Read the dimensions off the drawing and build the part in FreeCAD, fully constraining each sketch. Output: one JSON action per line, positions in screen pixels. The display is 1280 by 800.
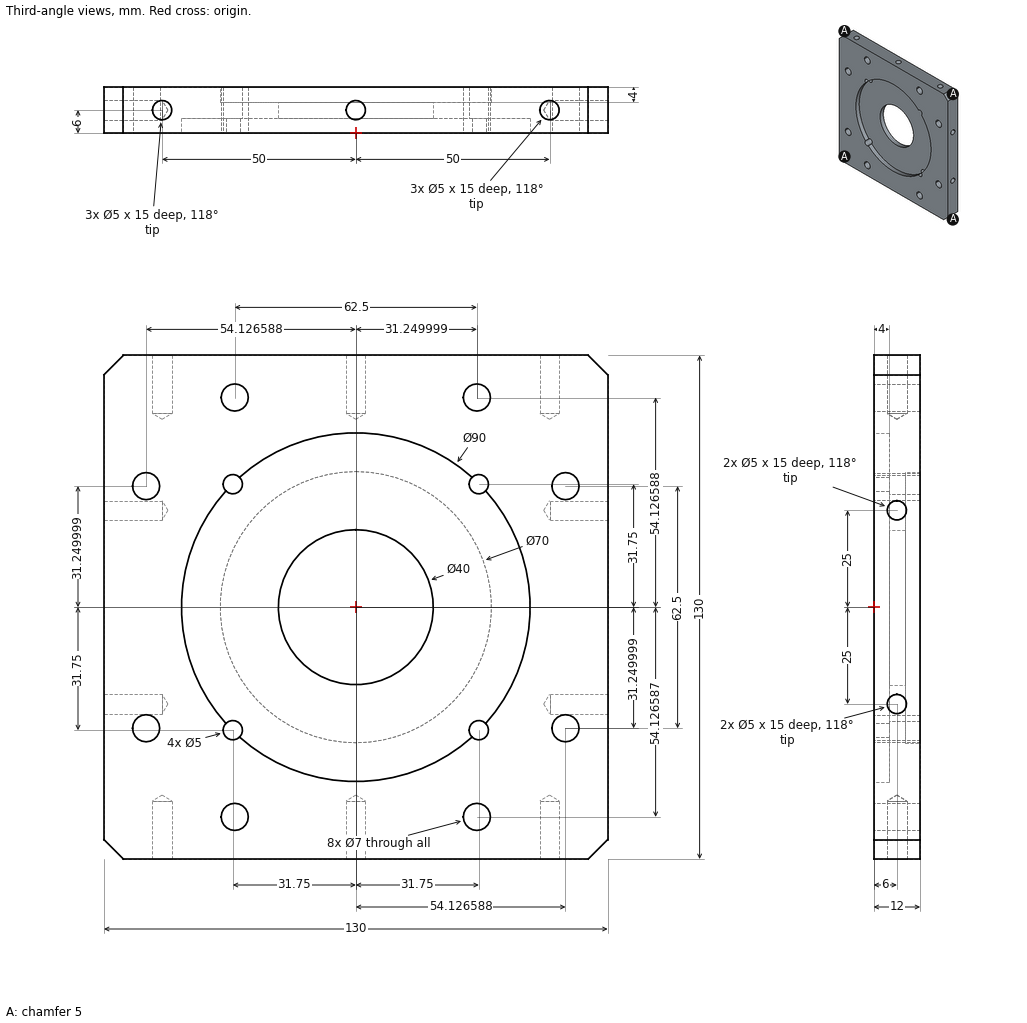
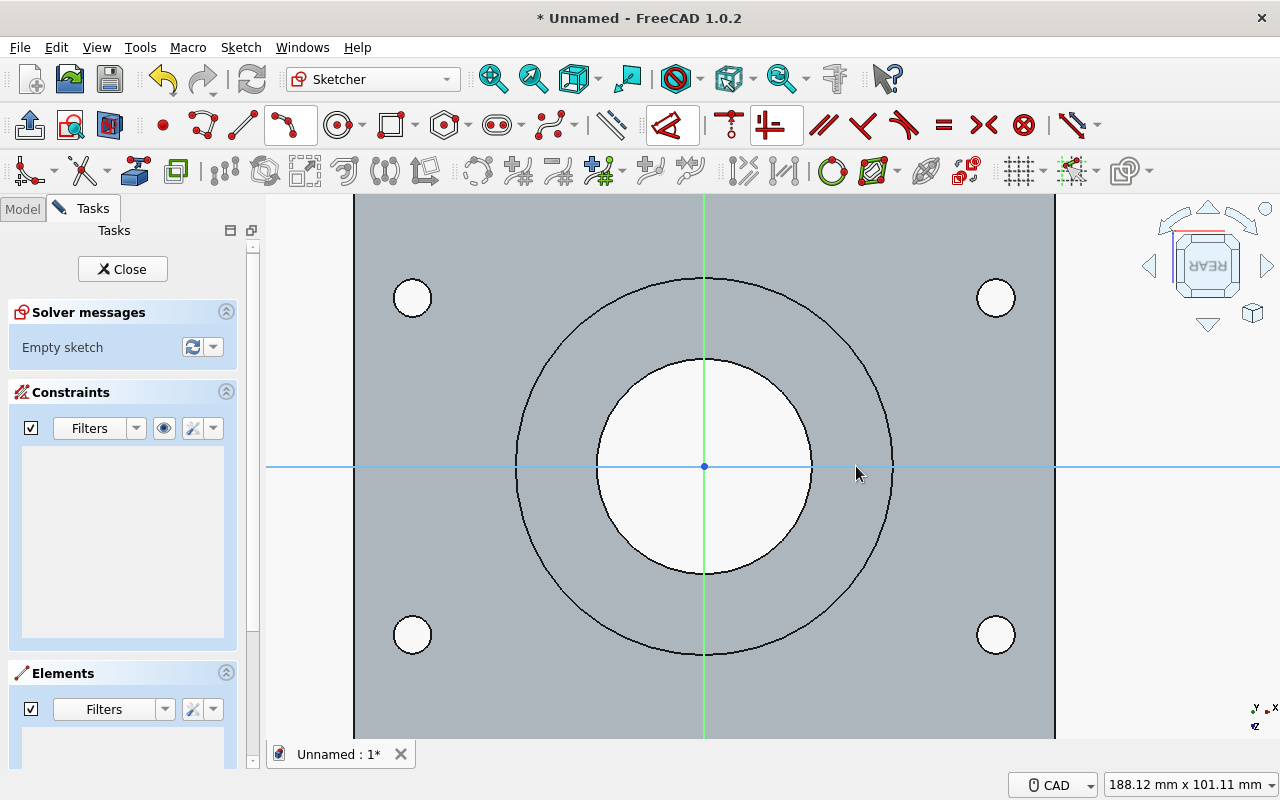
{"action": "key", "text": "g c"}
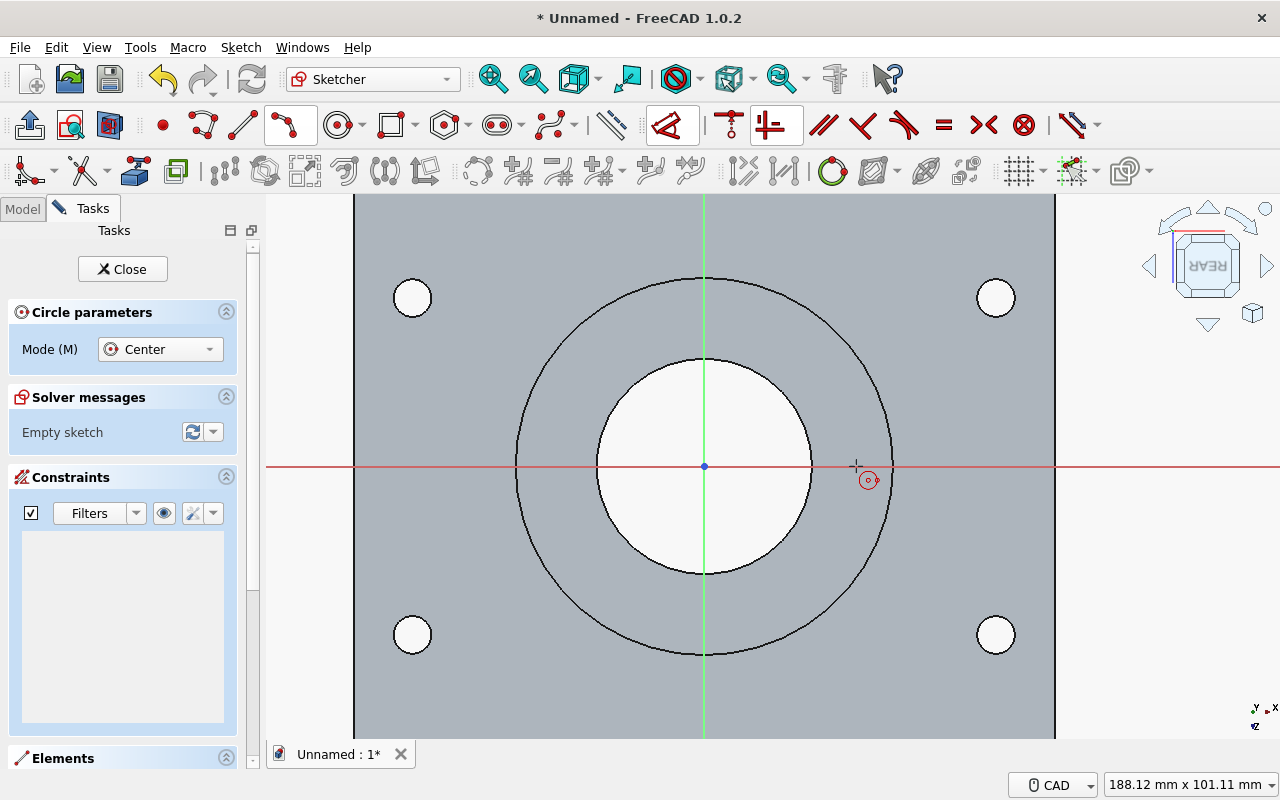
{"action": "scroll", "coordinate": [533, 295], "scroll_direction": "up", "scroll_amount": 3}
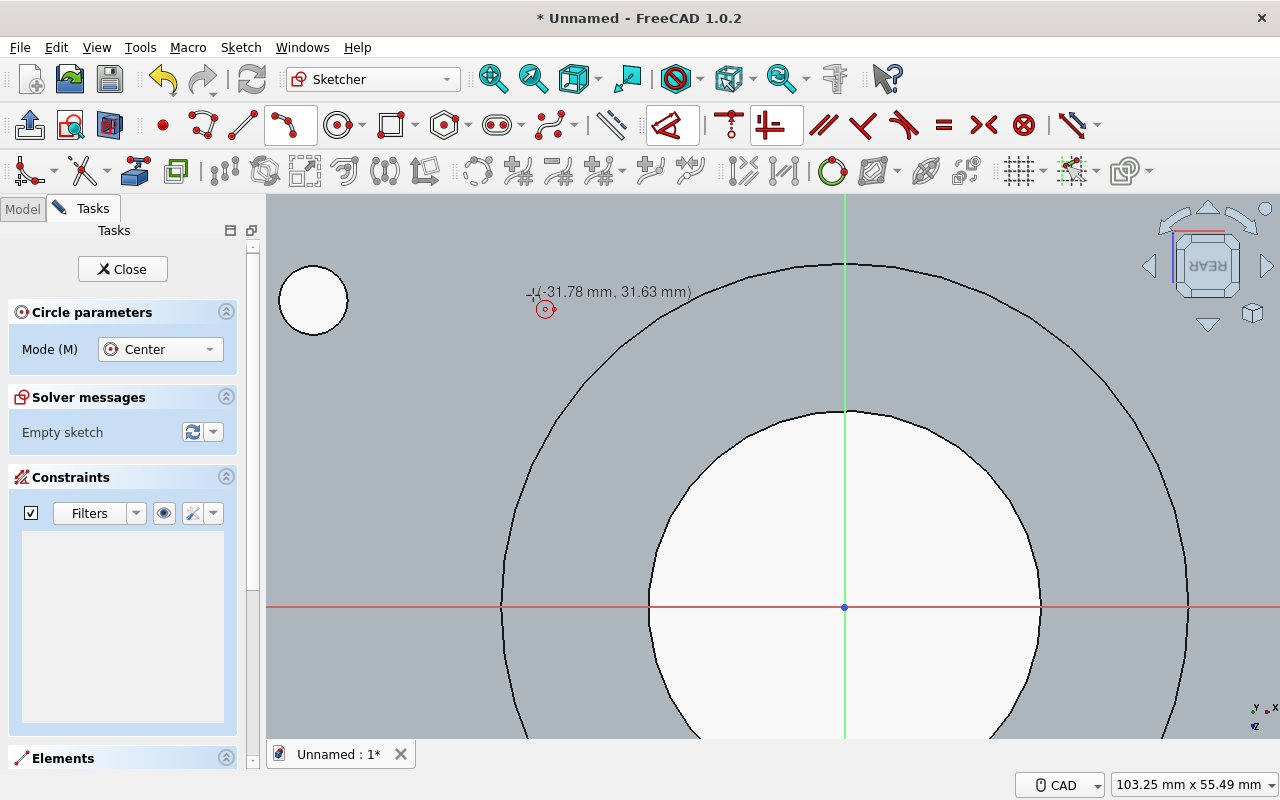
{"action": "left_click", "coordinate": [533, 296]}
{"action": "left_click", "coordinate": [550, 278]}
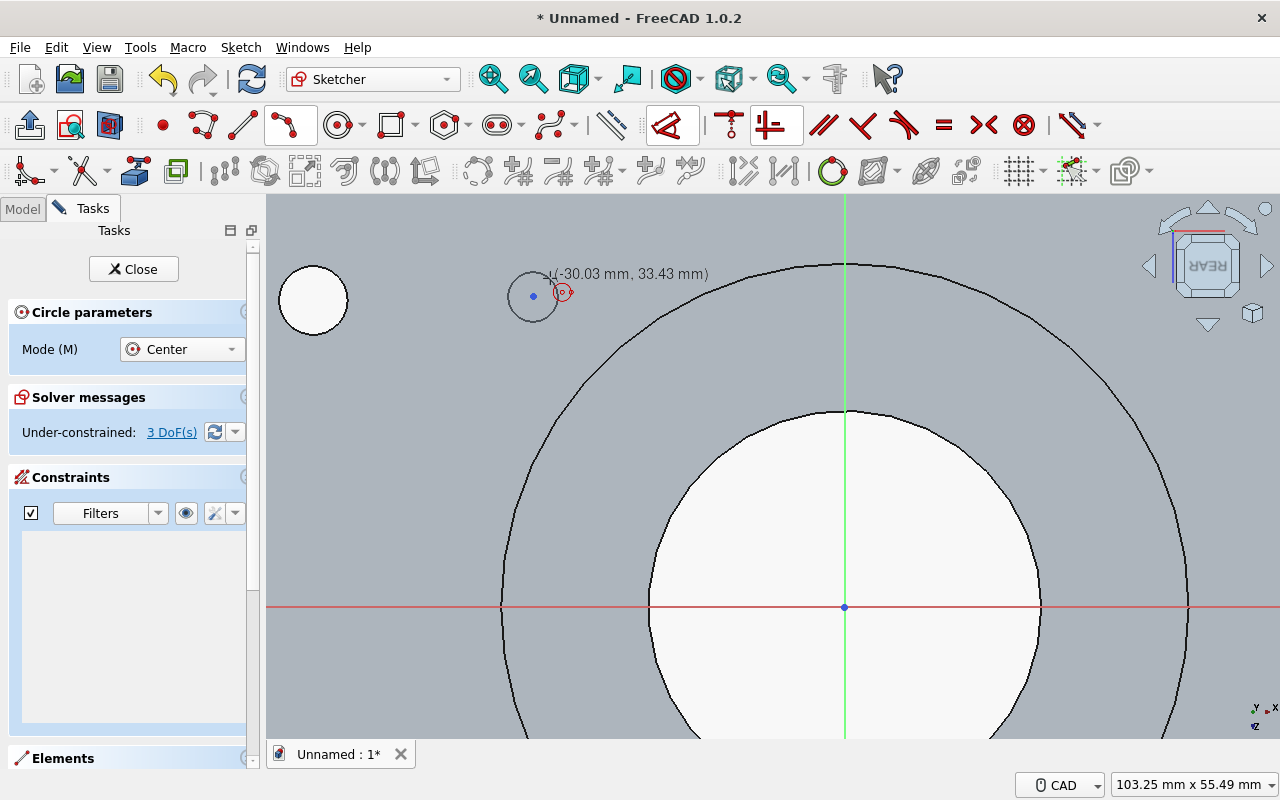
{"action": "scroll", "coordinate": [534, 295], "scroll_direction": "down", "scroll_amount": 3}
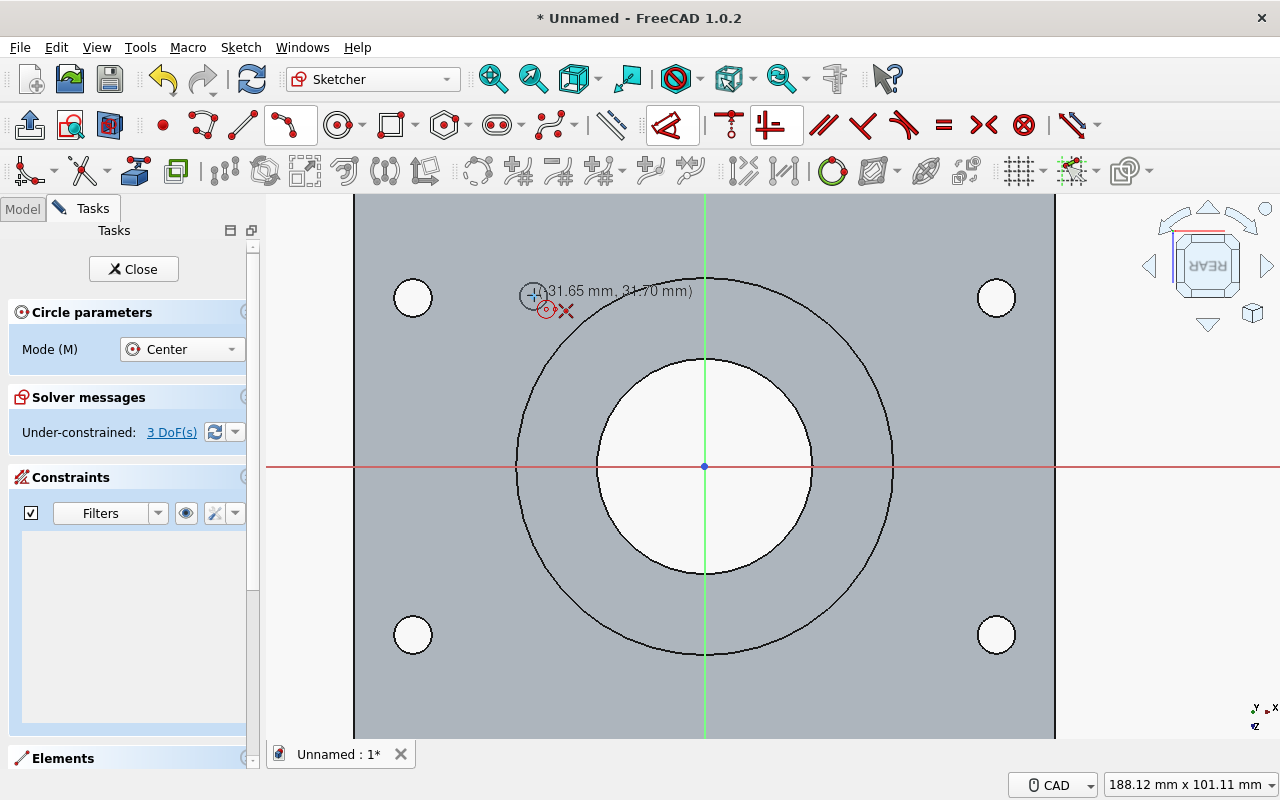
{"action": "scroll", "coordinate": [876, 295], "scroll_direction": "up", "scroll_amount": 3}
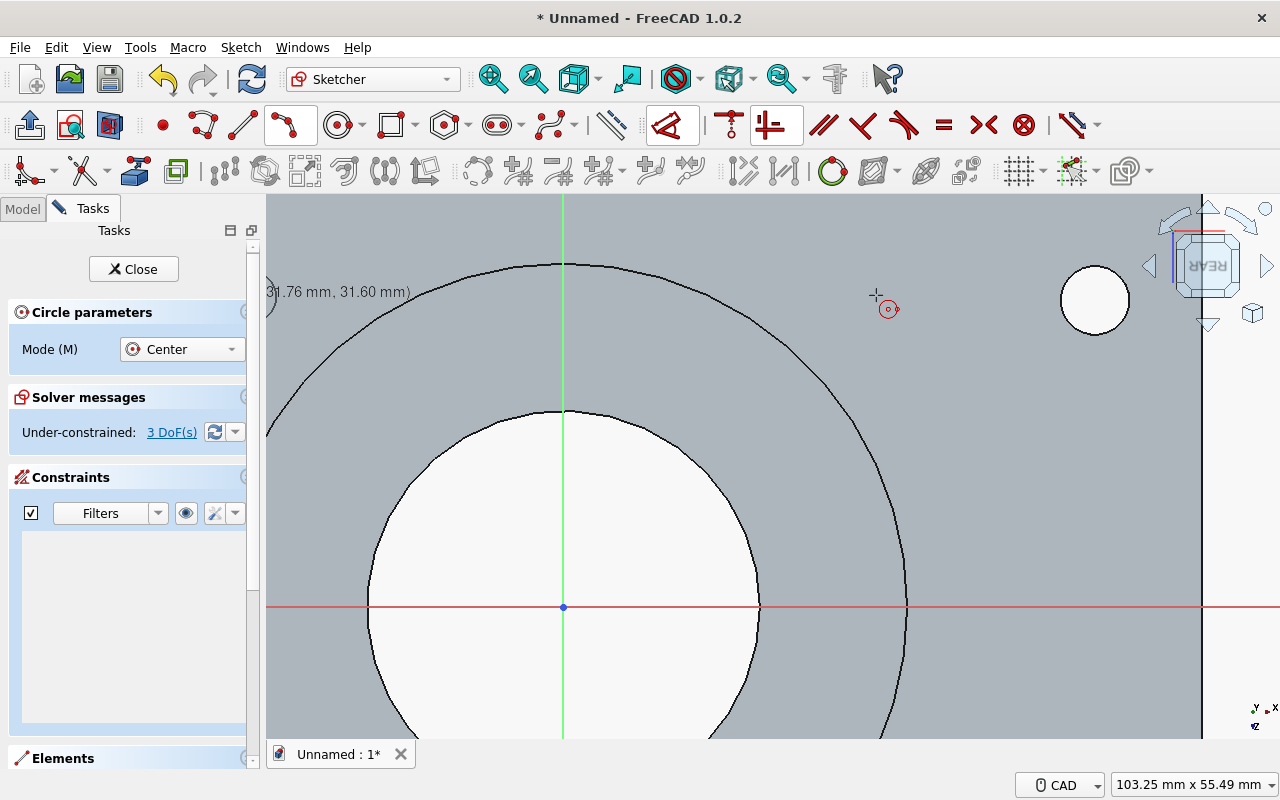
{"action": "left_click", "coordinate": [875, 296]}
{"action": "left_click", "coordinate": [893, 278]}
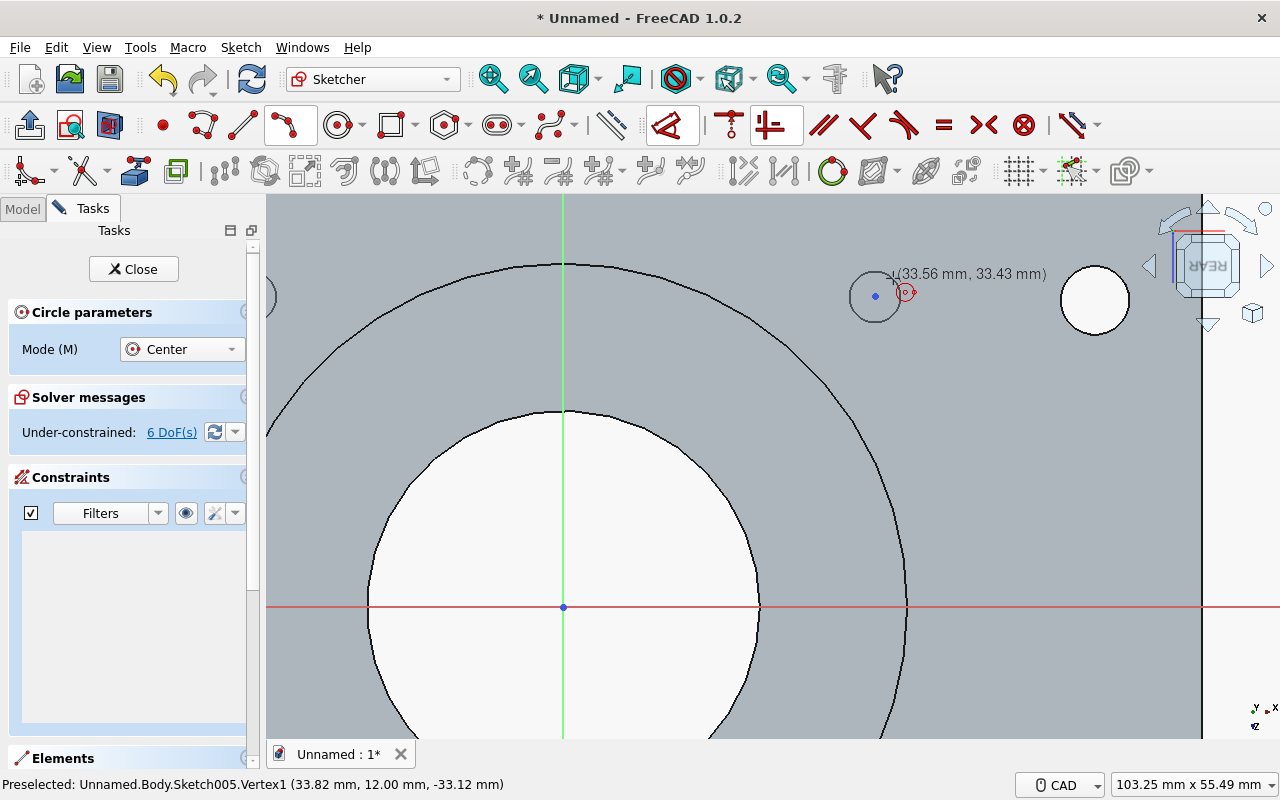
{"action": "scroll", "coordinate": [876, 295], "scroll_direction": "down", "scroll_amount": 3}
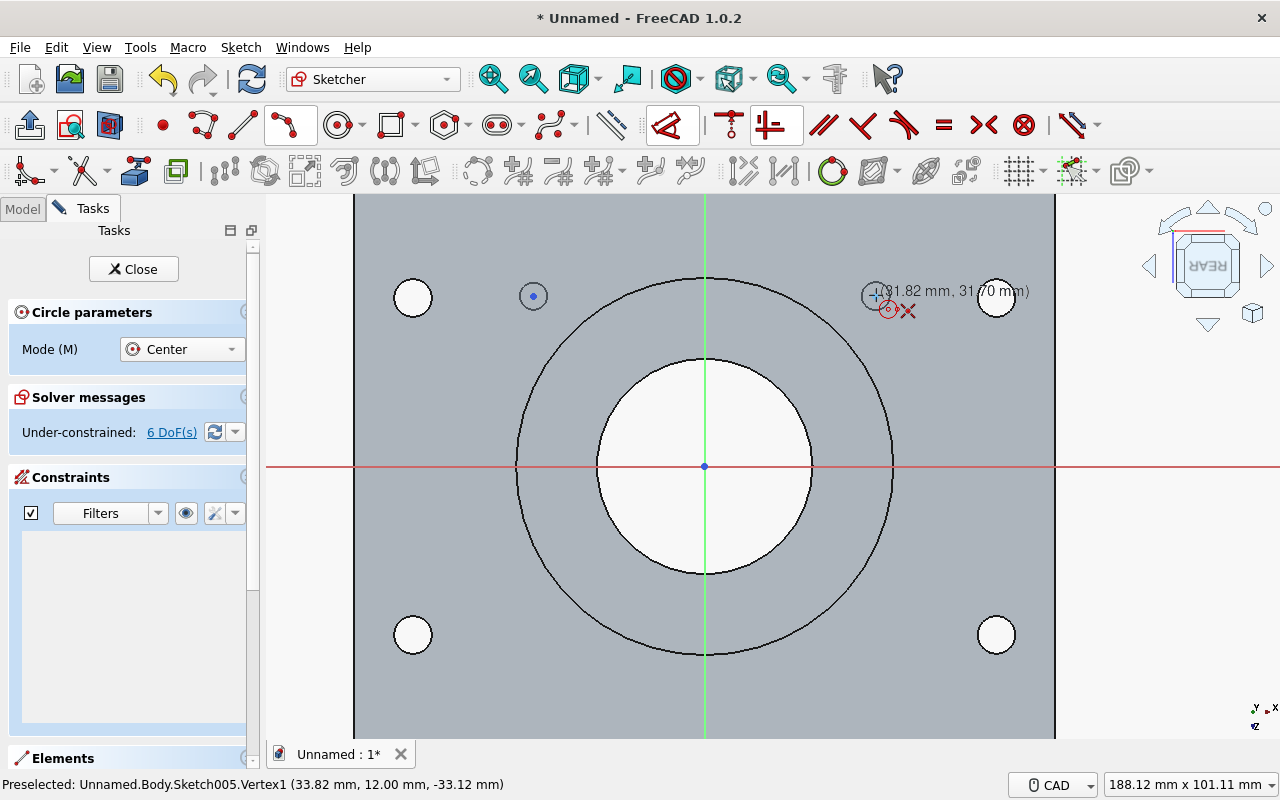
{"action": "scroll", "coordinate": [876, 638], "scroll_direction": "up", "scroll_amount": 3}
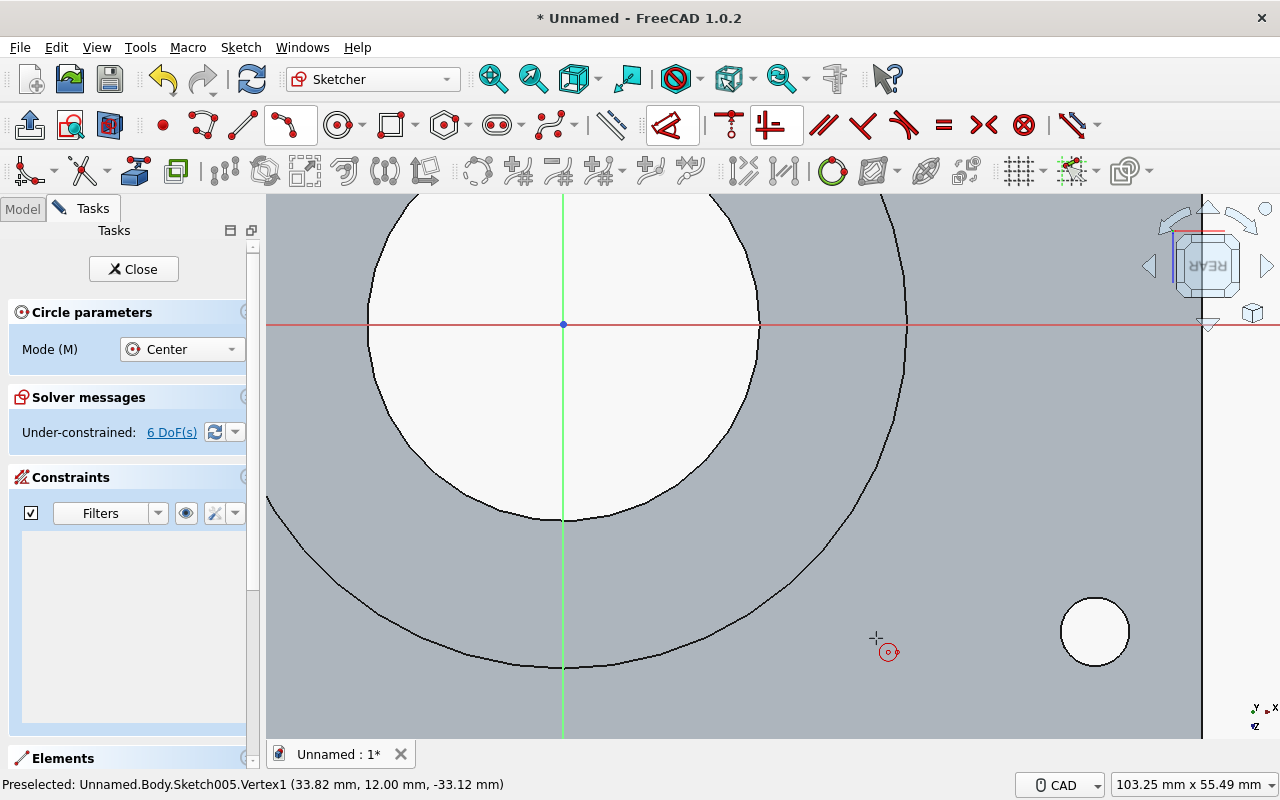
{"action": "left_click", "coordinate": [875, 637]}
{"action": "left_click", "coordinate": [893, 619]}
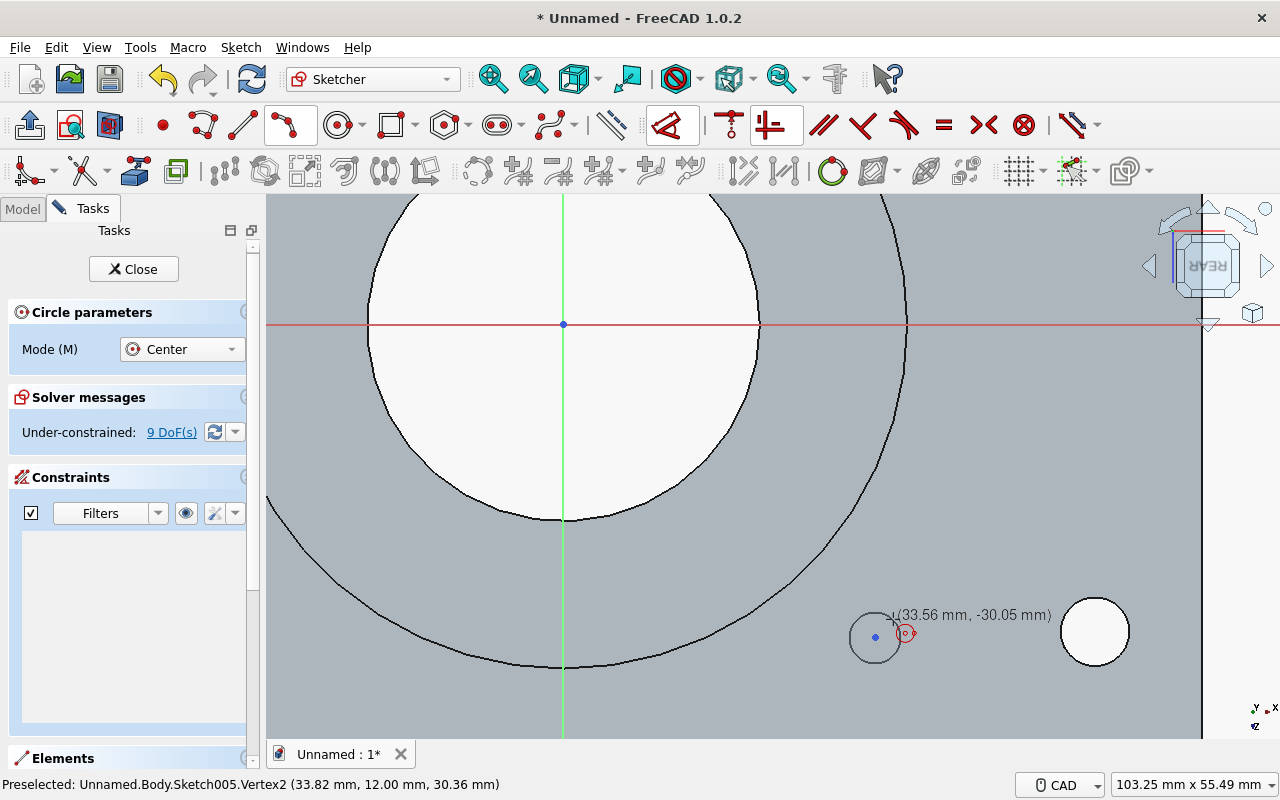
{"action": "scroll", "coordinate": [876, 639], "scroll_direction": "down", "scroll_amount": 3}